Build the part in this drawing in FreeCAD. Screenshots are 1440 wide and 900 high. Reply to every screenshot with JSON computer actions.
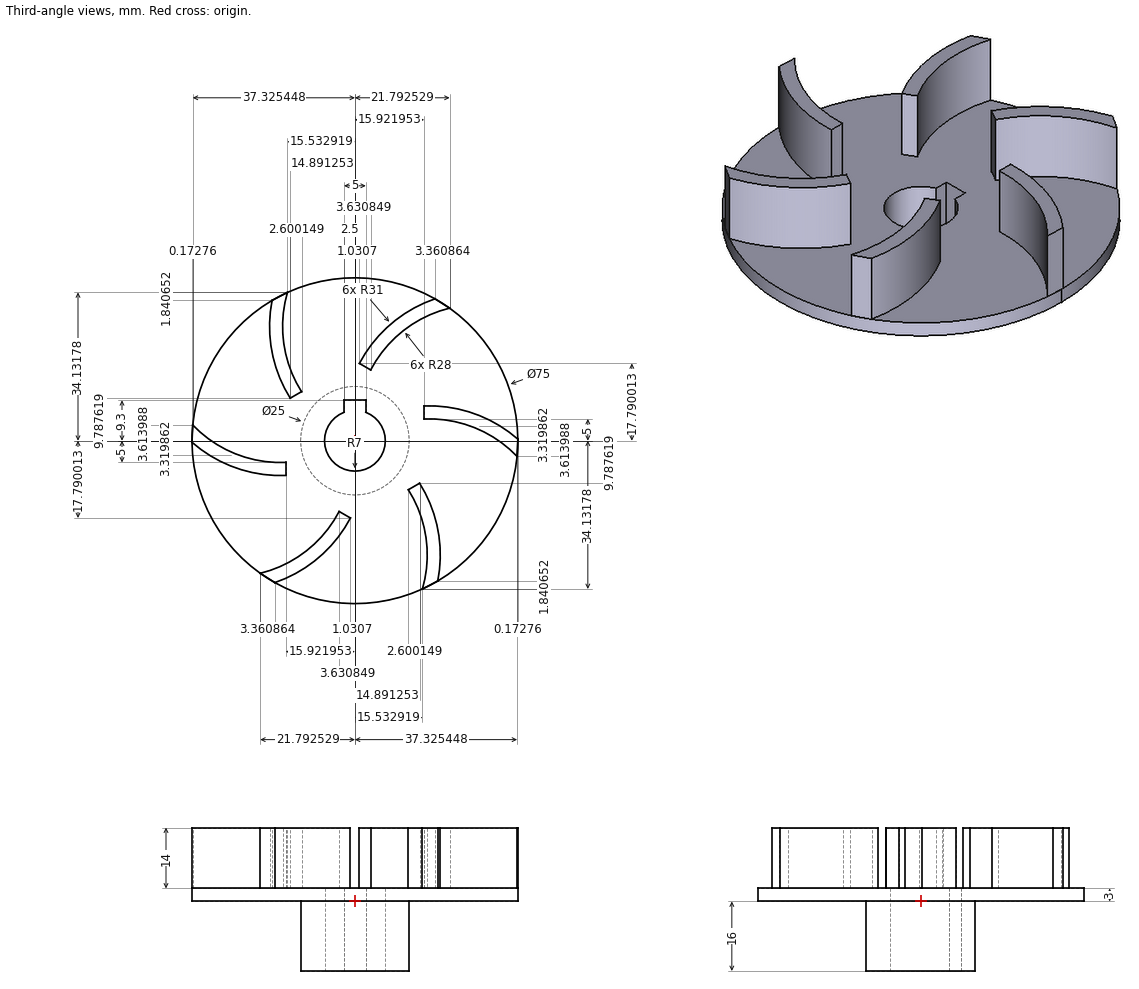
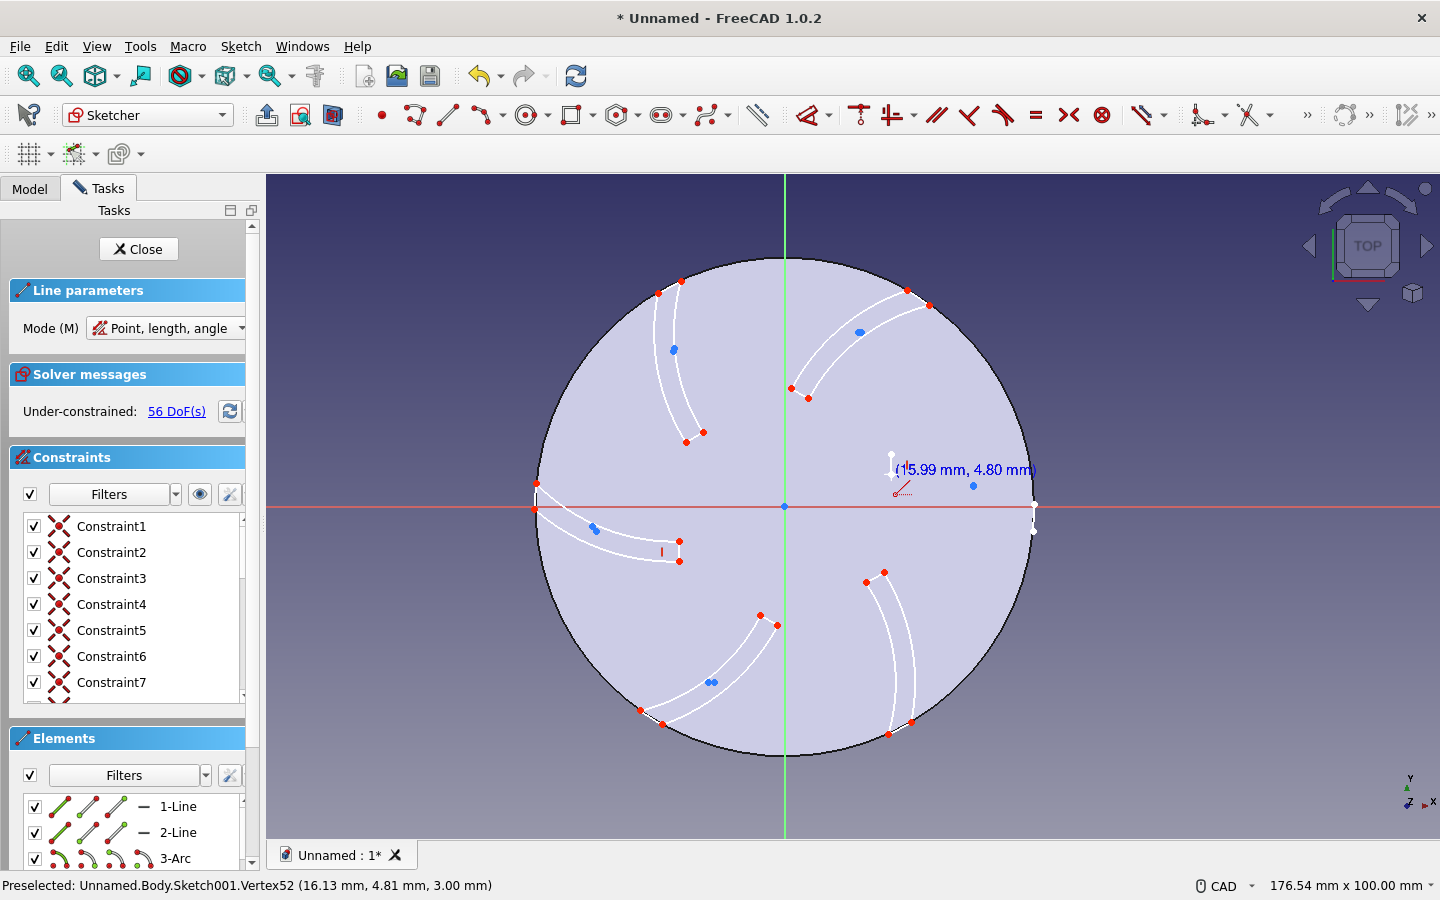
{"action": "key", "text": "g 3 a"}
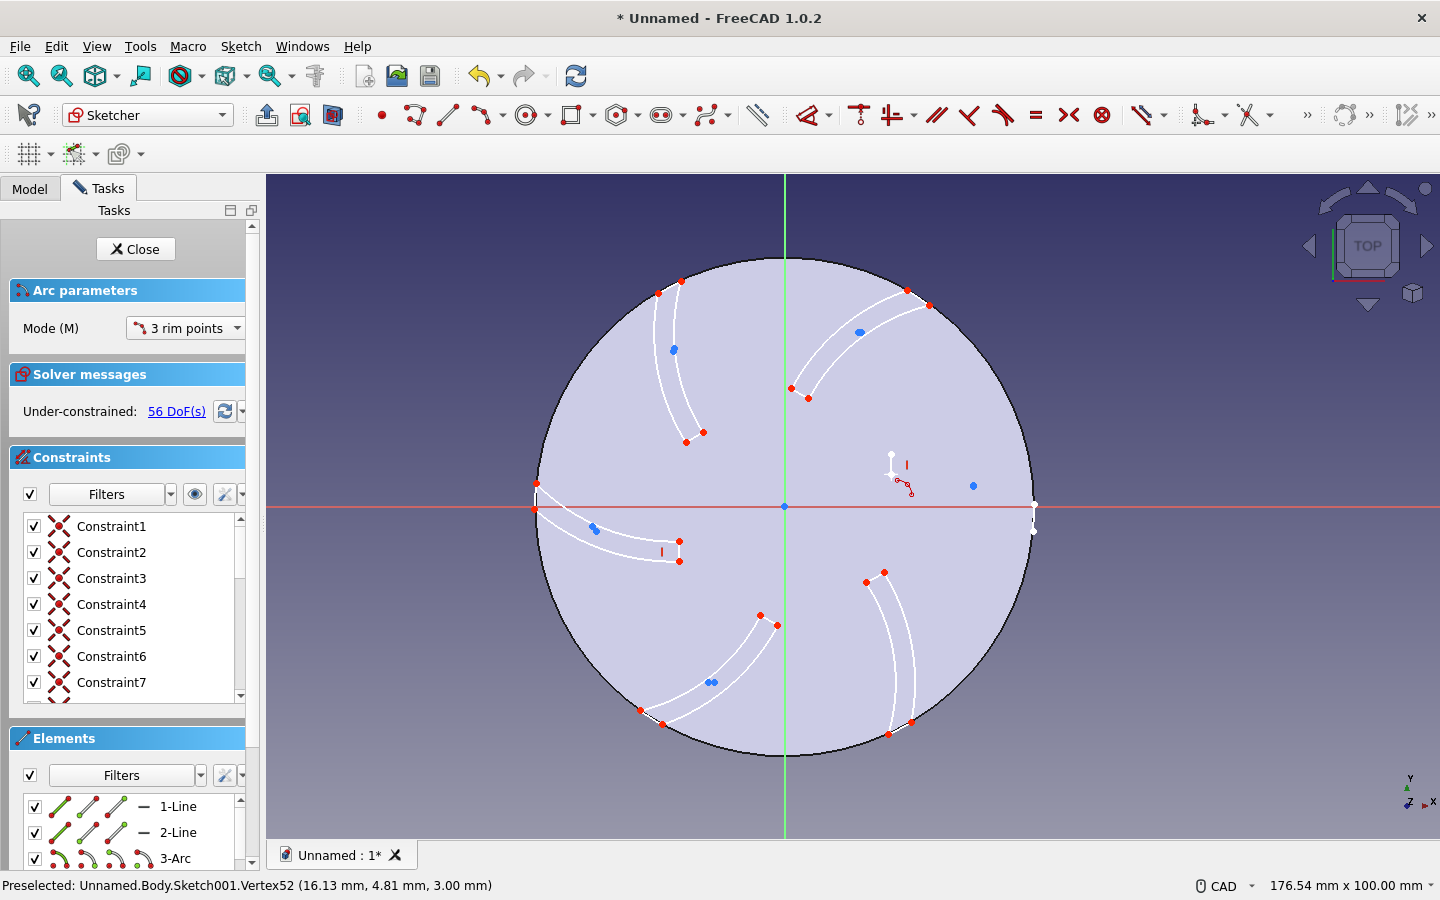
{"action": "scroll", "coordinate": [1034, 504], "scroll_direction": "up", "scroll_amount": 10}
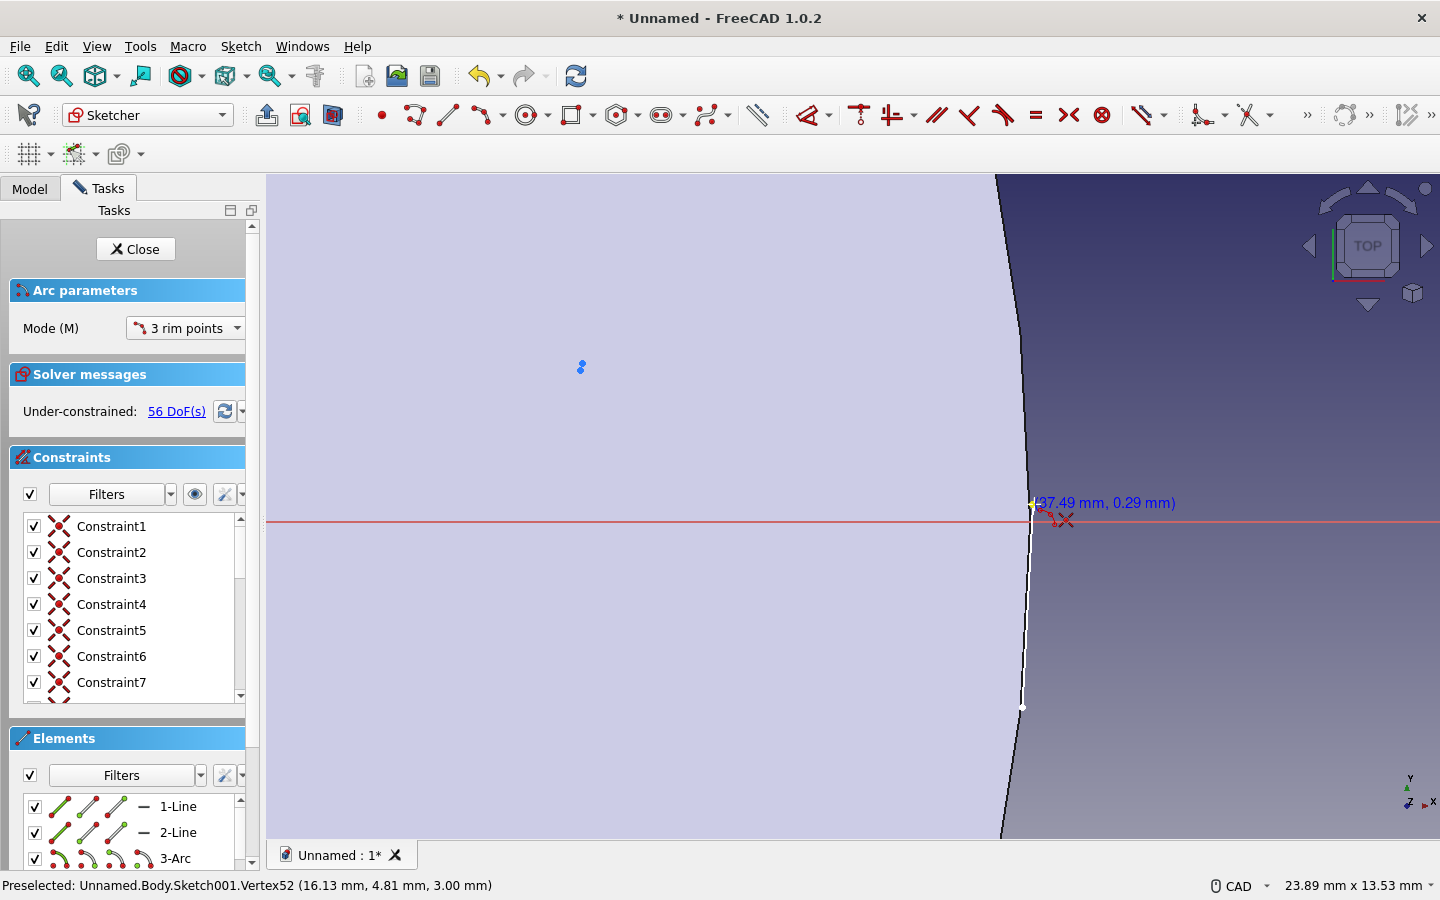
{"action": "left_click", "coordinate": [1033, 505]}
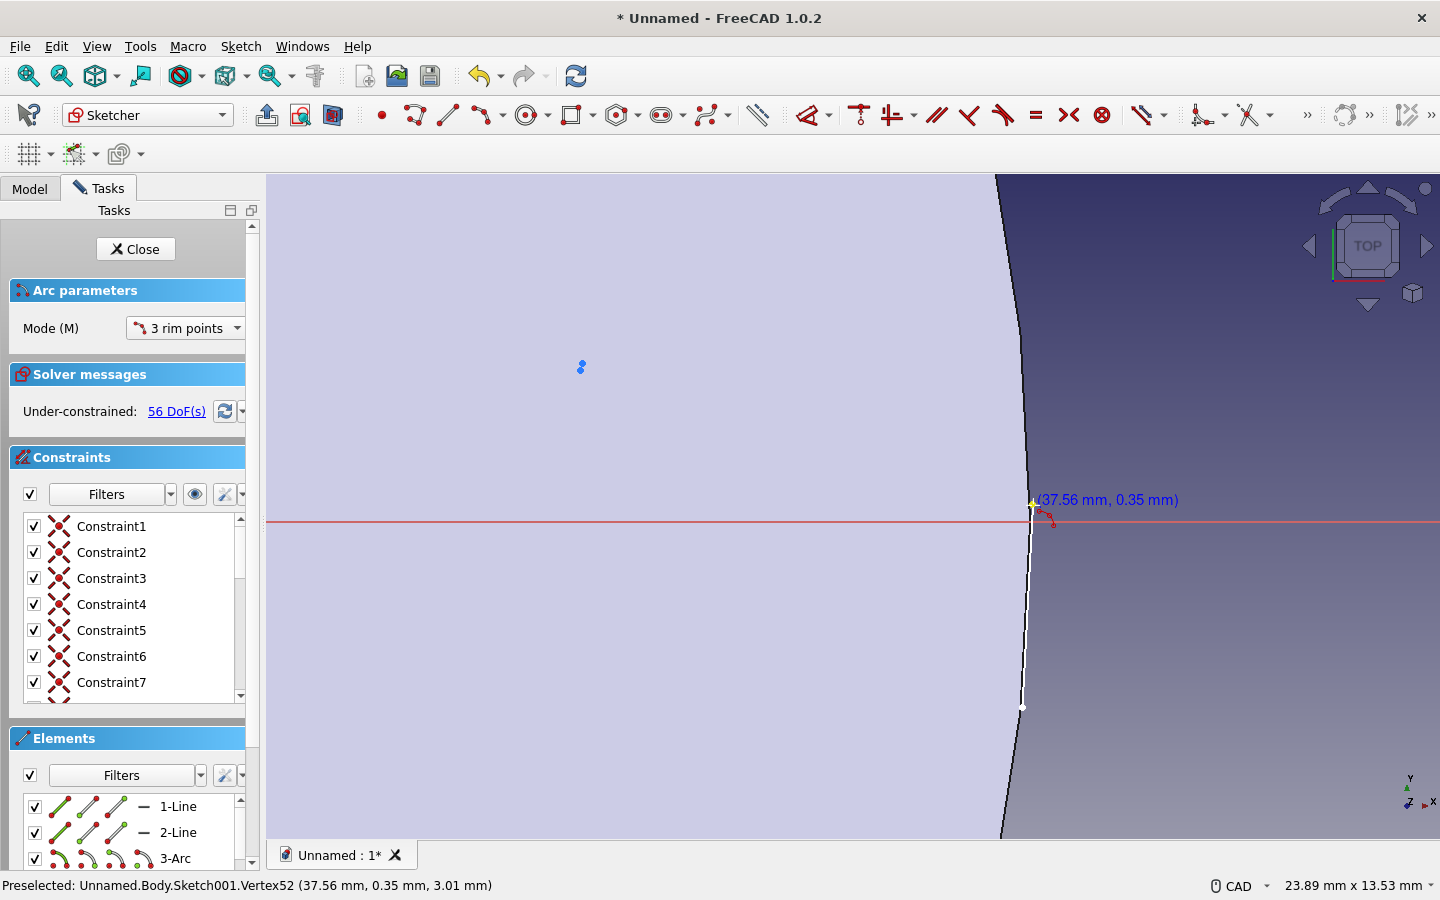
{"action": "scroll", "coordinate": [1034, 504], "scroll_direction": "down", "scroll_amount": 10}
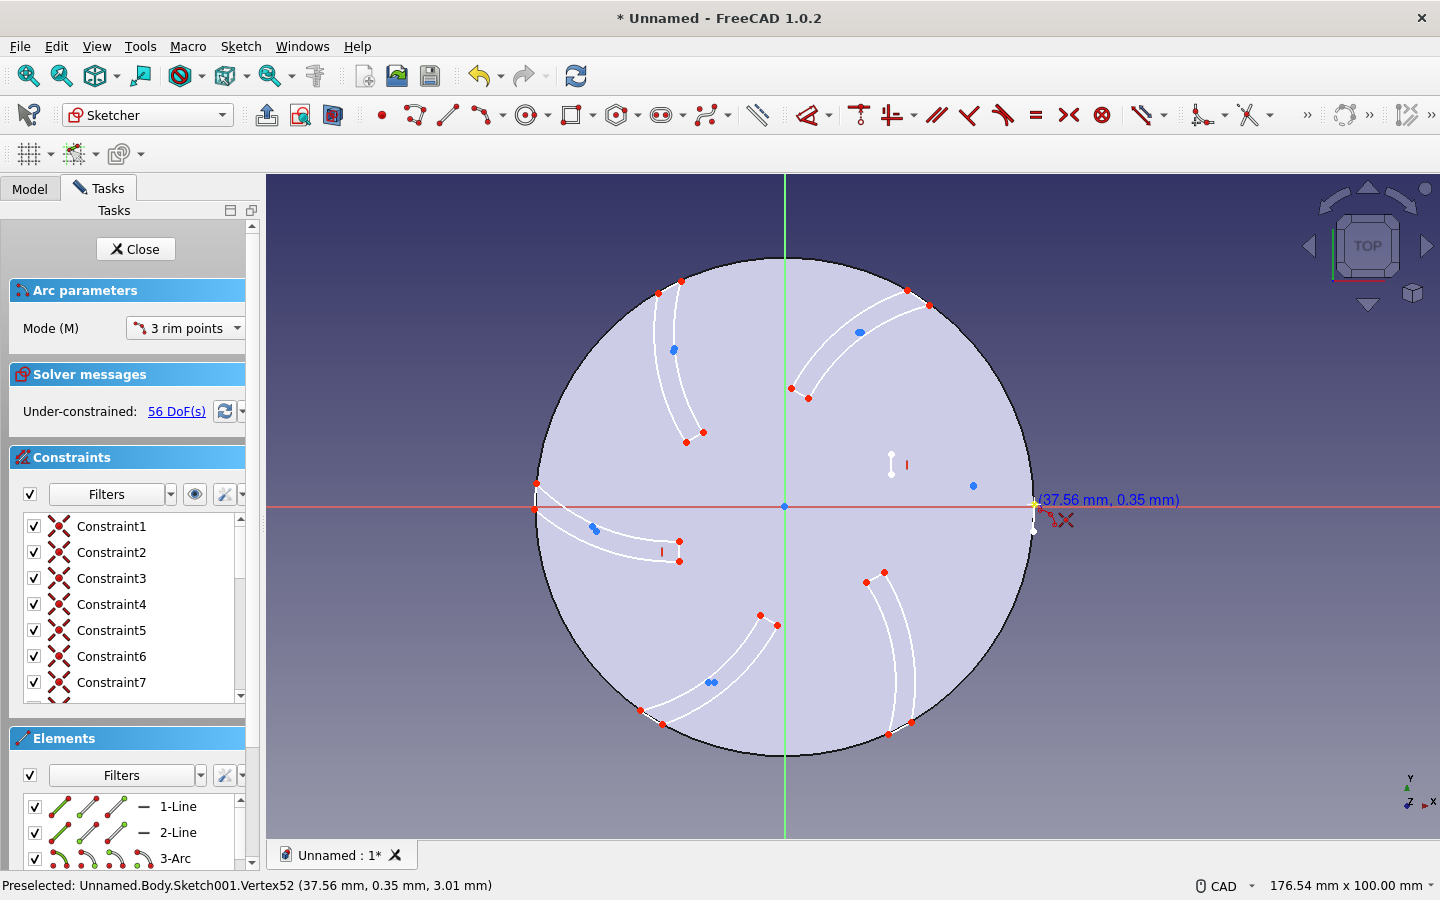
{"action": "scroll", "coordinate": [891, 454], "scroll_direction": "up", "scroll_amount": 3}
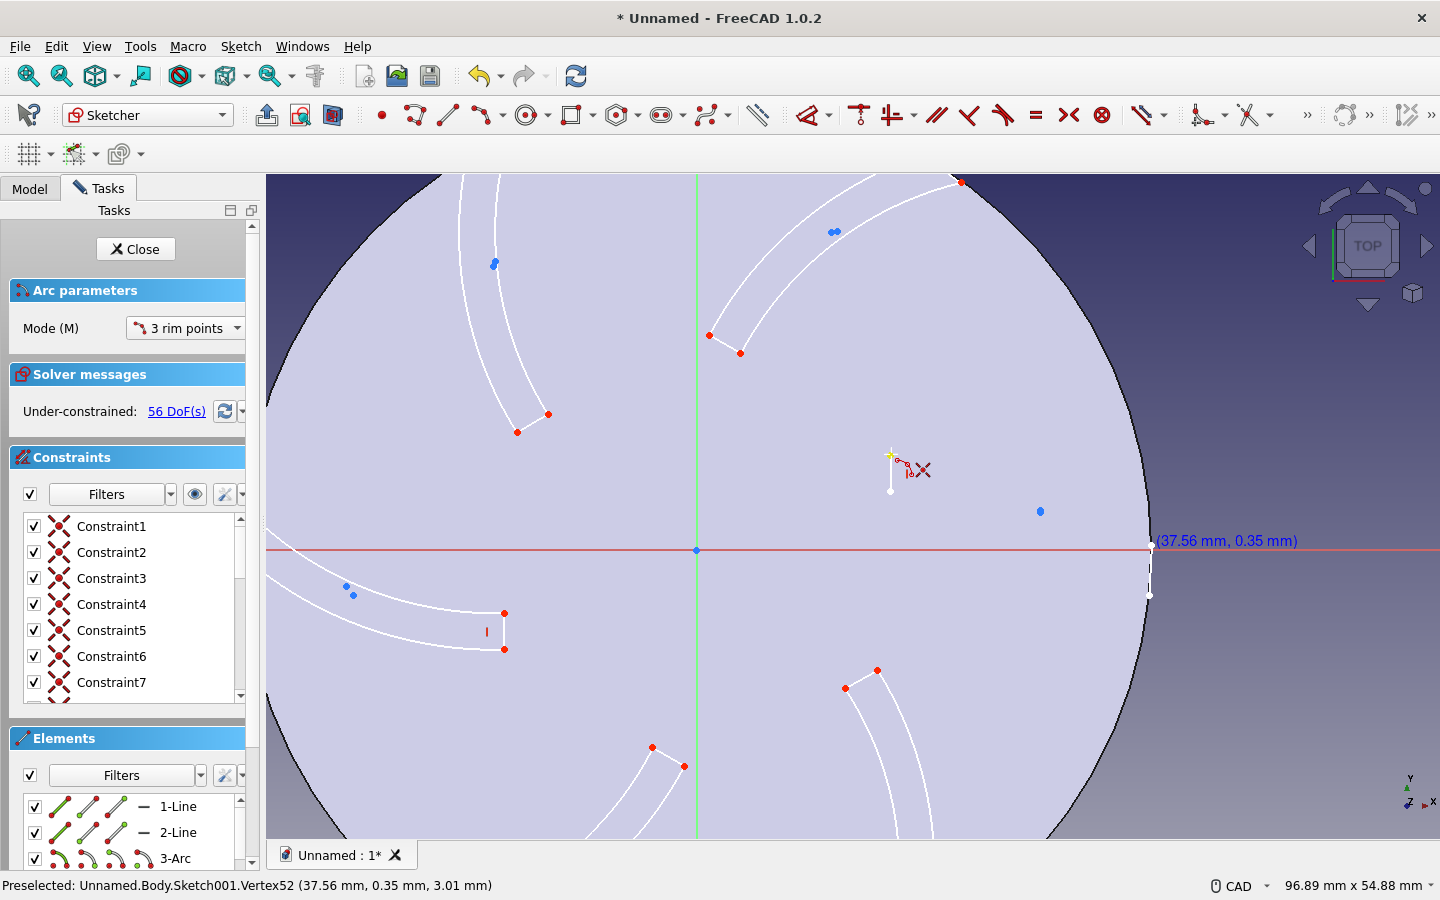
{"action": "left_click", "coordinate": [891, 455]}
{"action": "left_click", "coordinate": [1029, 474]}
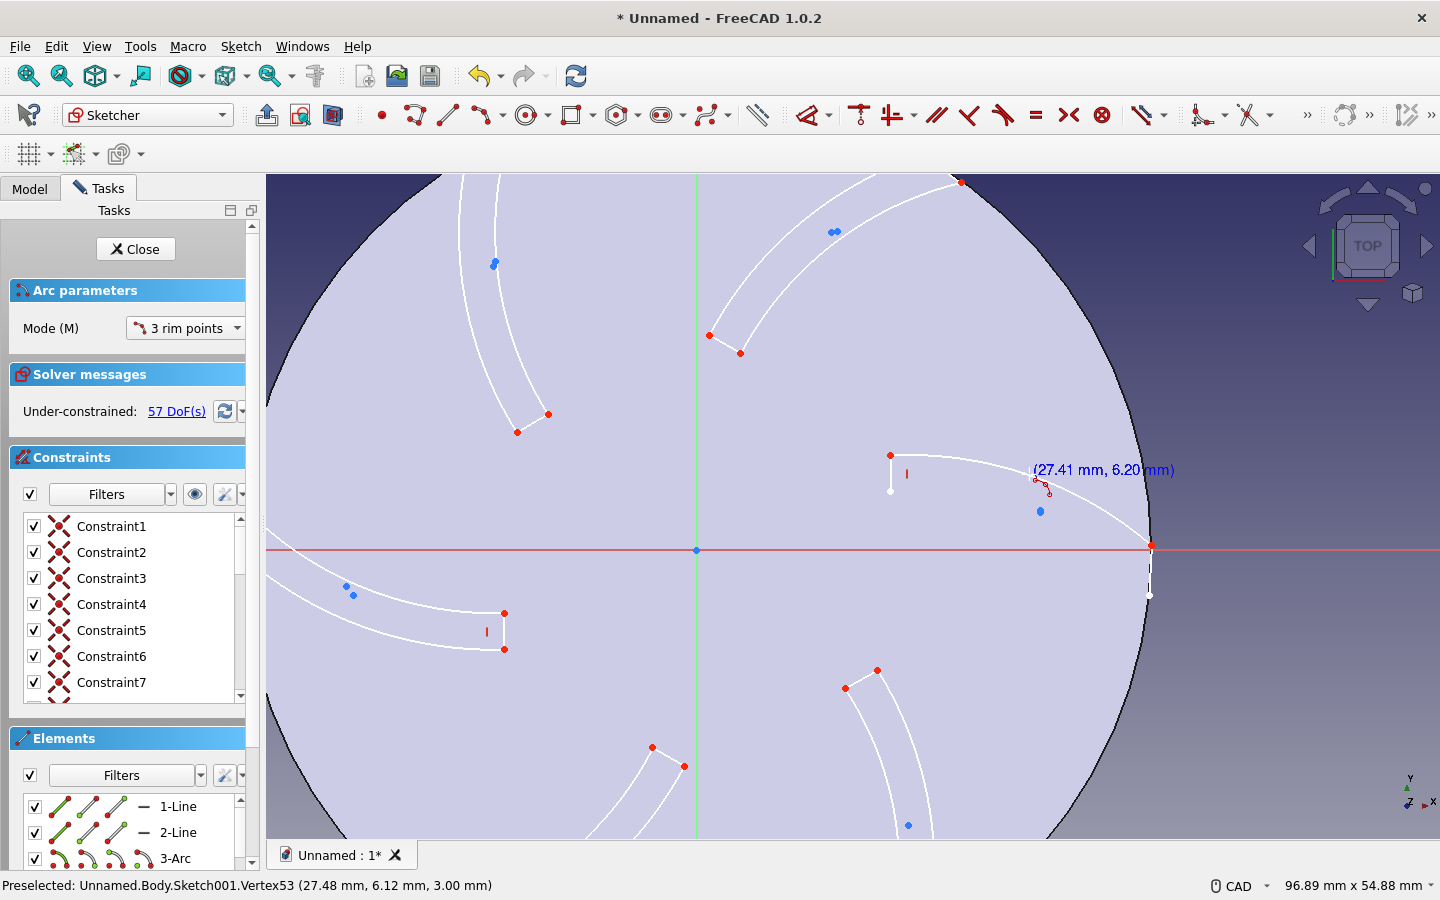
{"action": "left_click", "coordinate": [891, 492]}
{"action": "left_click", "coordinate": [1149, 596]}
{"action": "left_click", "coordinate": [1004, 504]}
{"action": "key", "text": "Escape"}